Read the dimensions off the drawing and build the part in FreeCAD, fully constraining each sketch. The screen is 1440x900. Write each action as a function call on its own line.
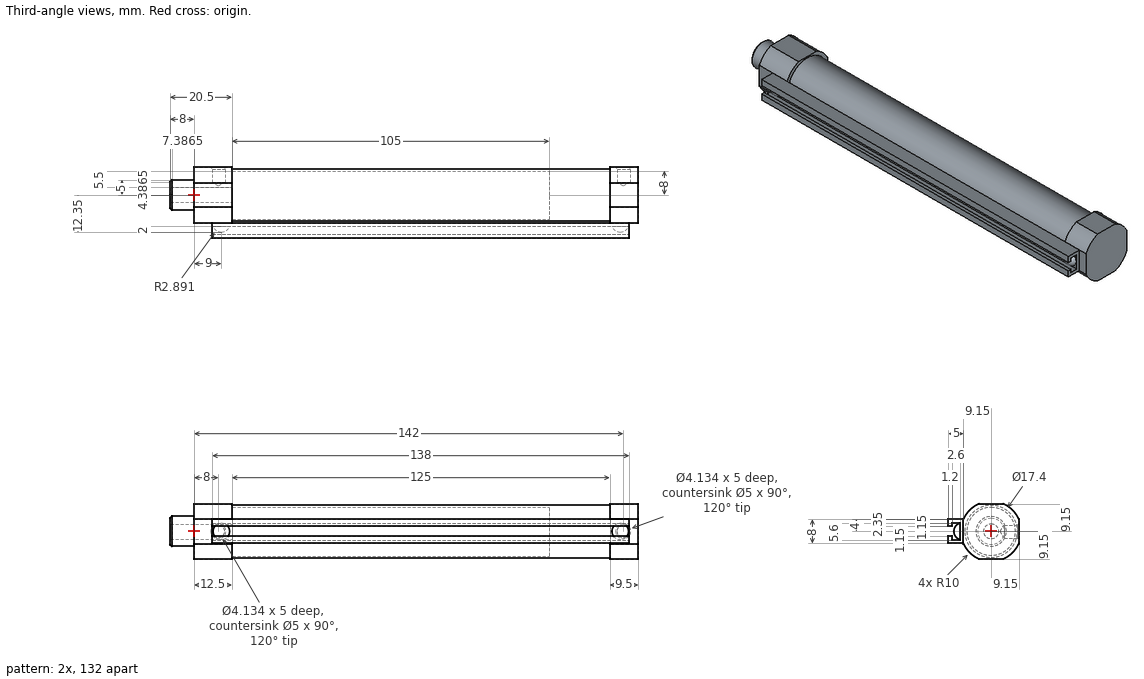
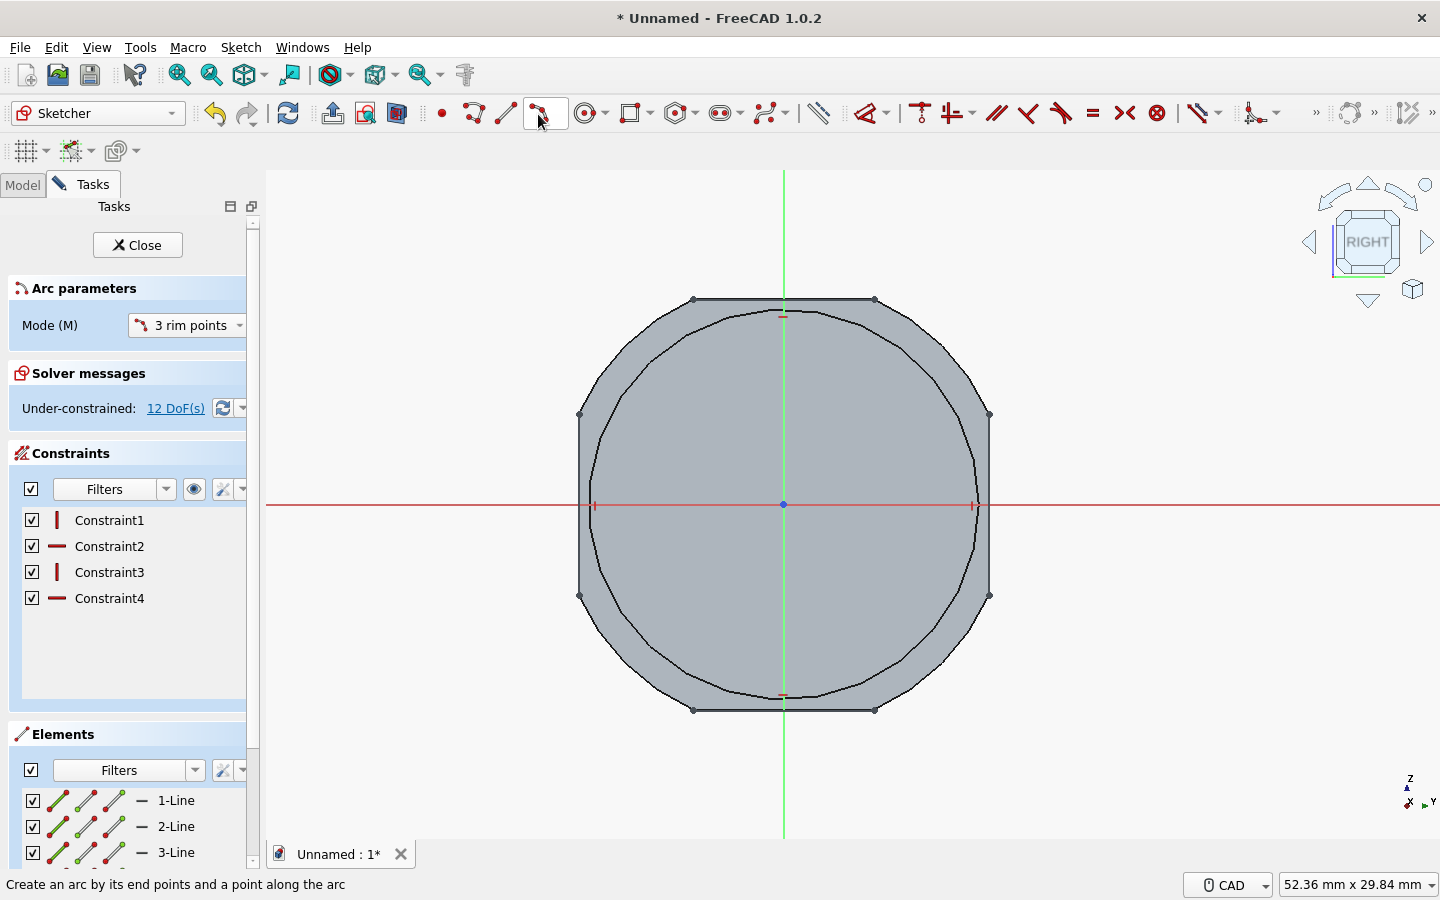
click(579, 596)
click(693, 711)
click(625, 663)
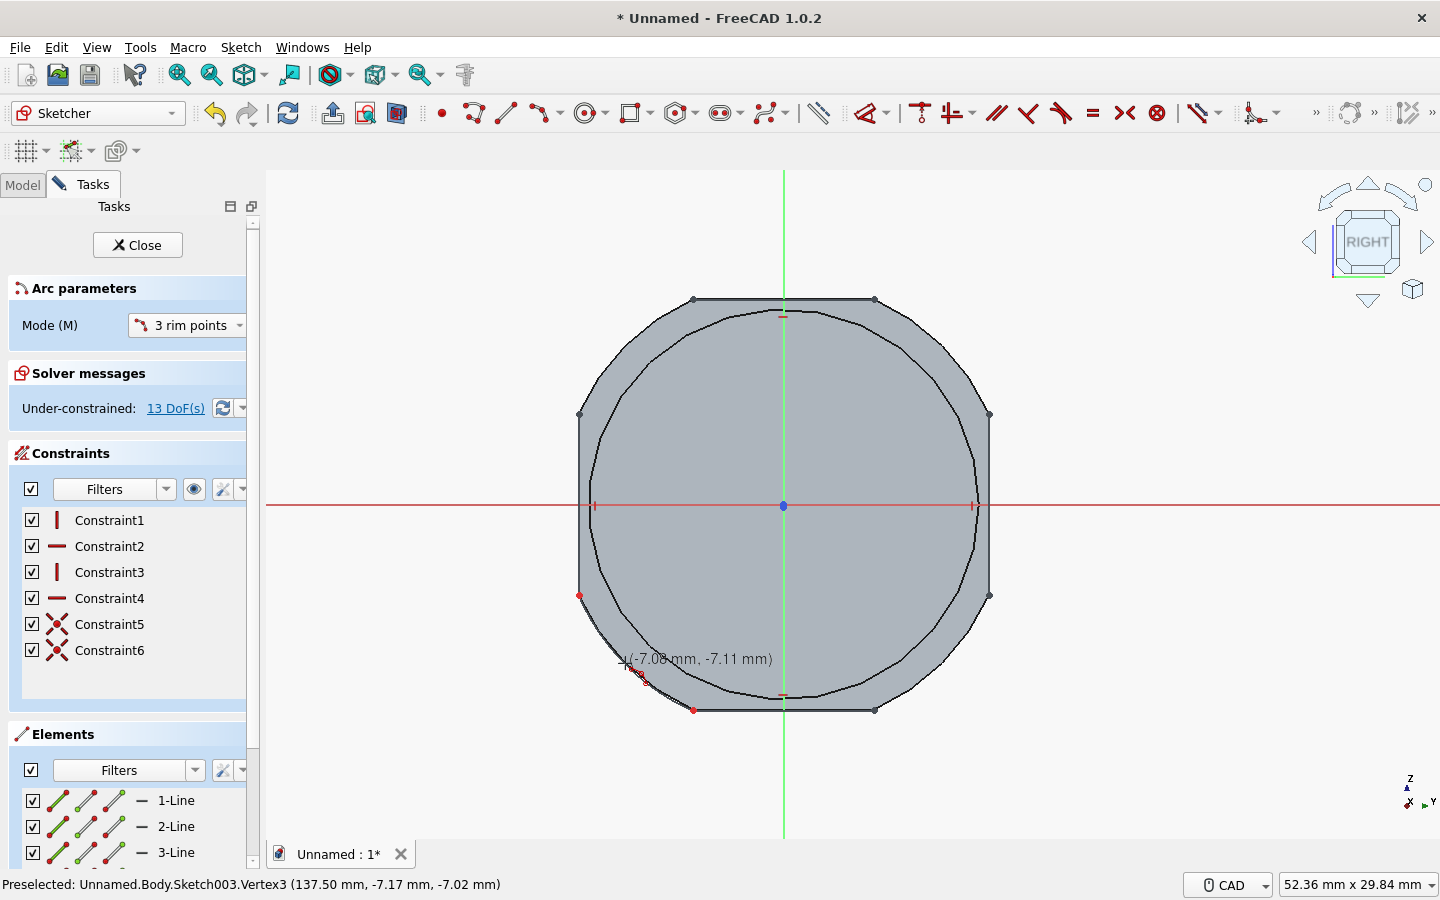
click(874, 711)
click(989, 596)
click(942, 663)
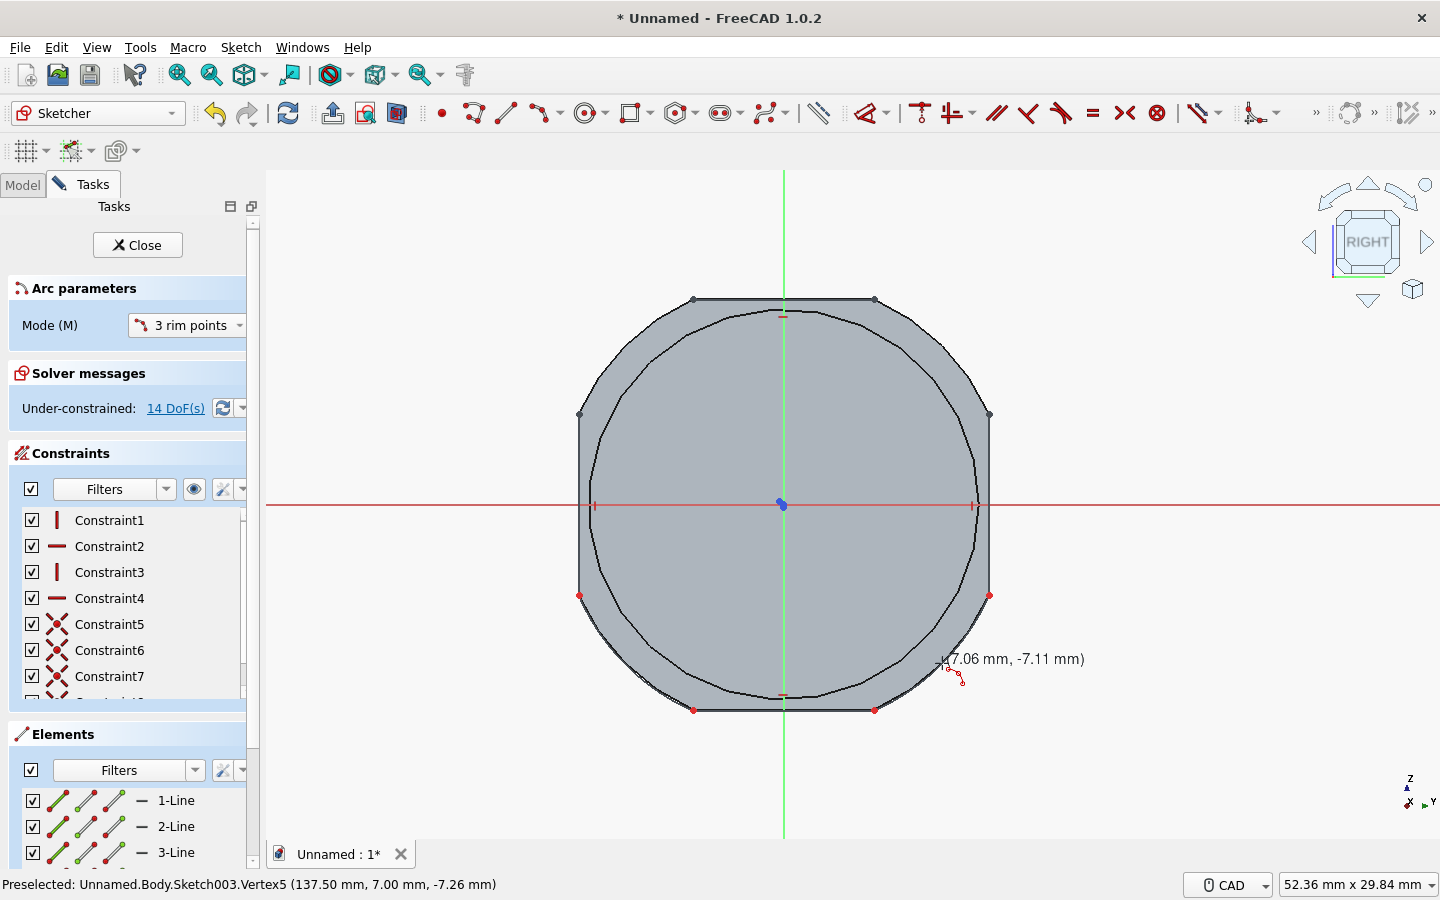
click(989, 415)
click(874, 300)
click(942, 346)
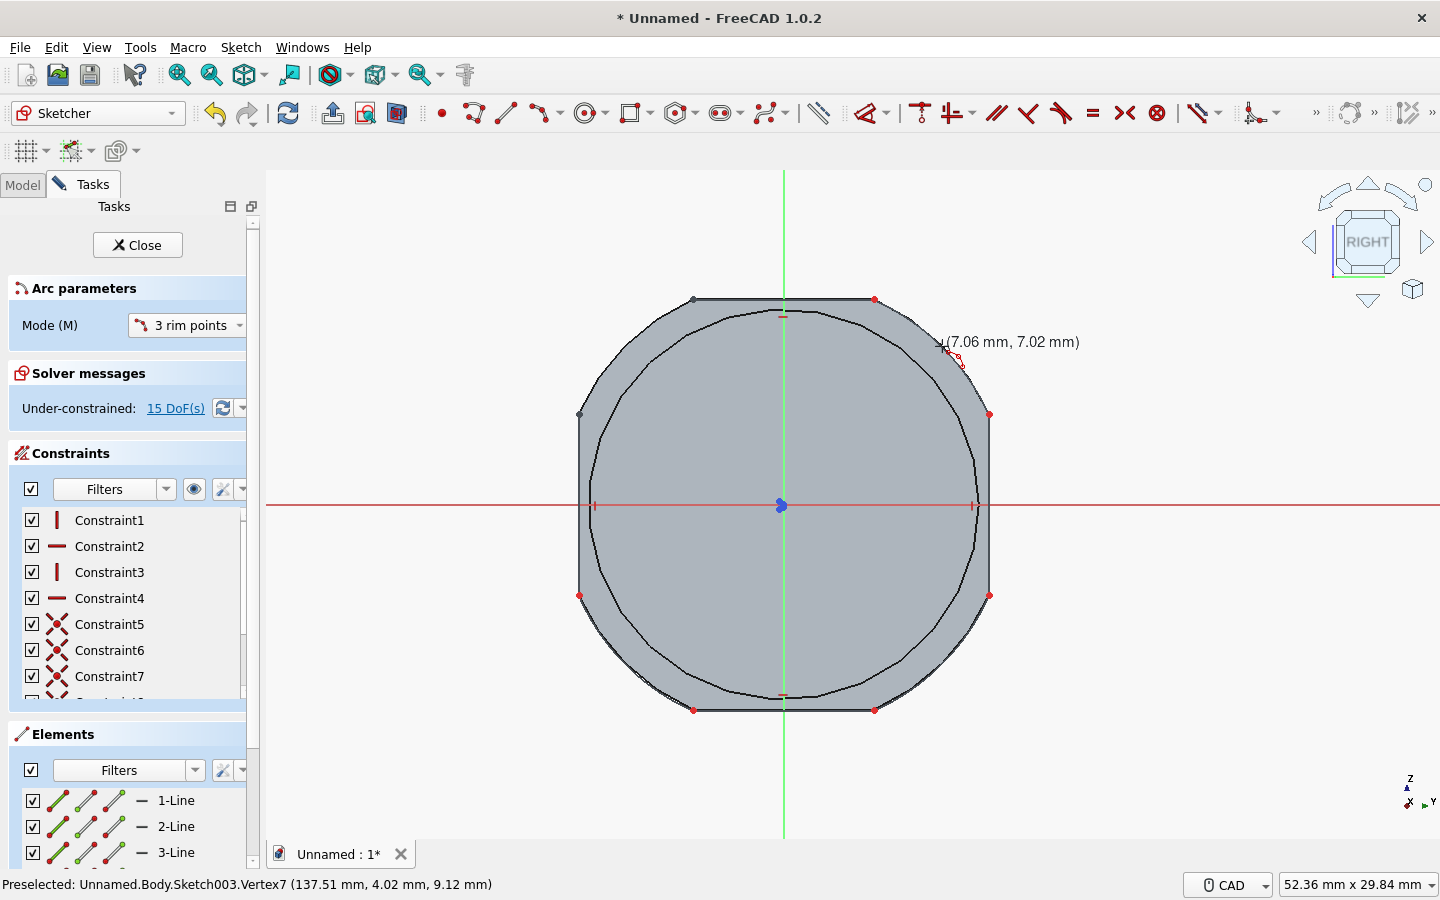
click(693, 300)
click(579, 415)
click(625, 346)
key(Escape)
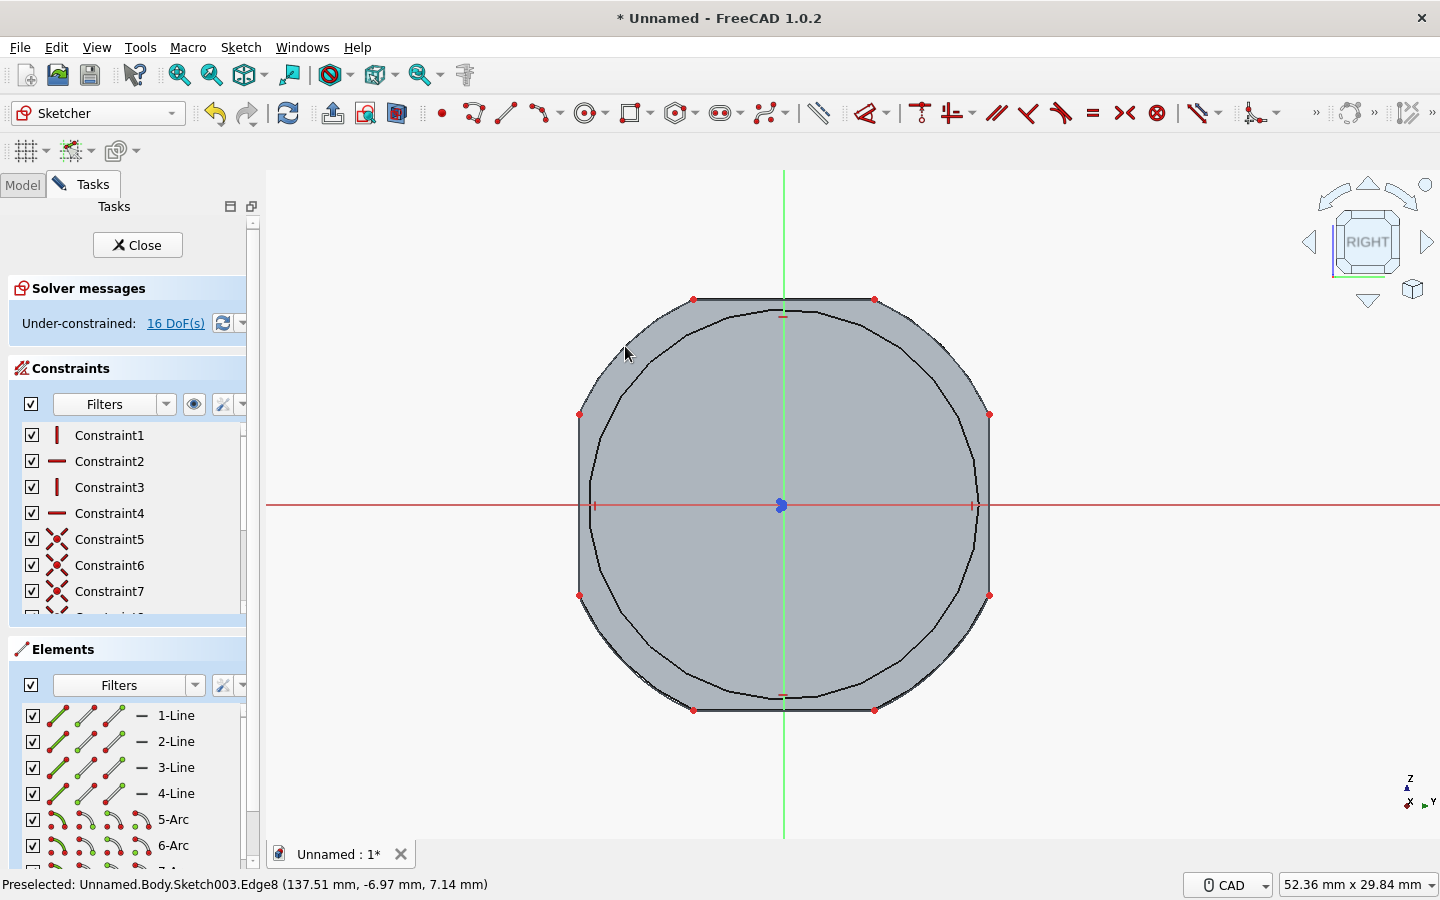
click(604, 639)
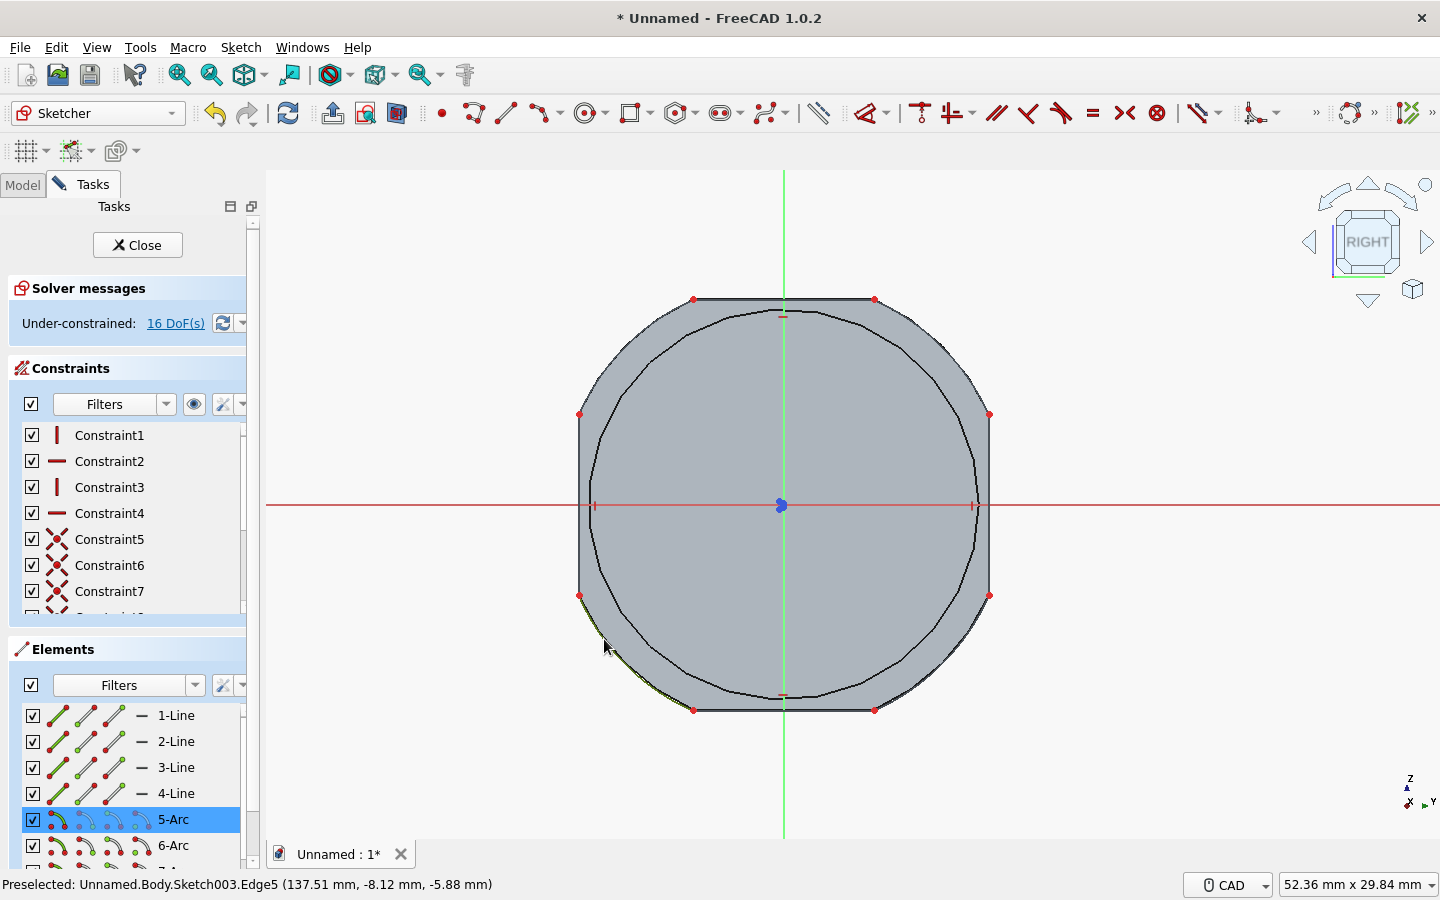
click(917, 686)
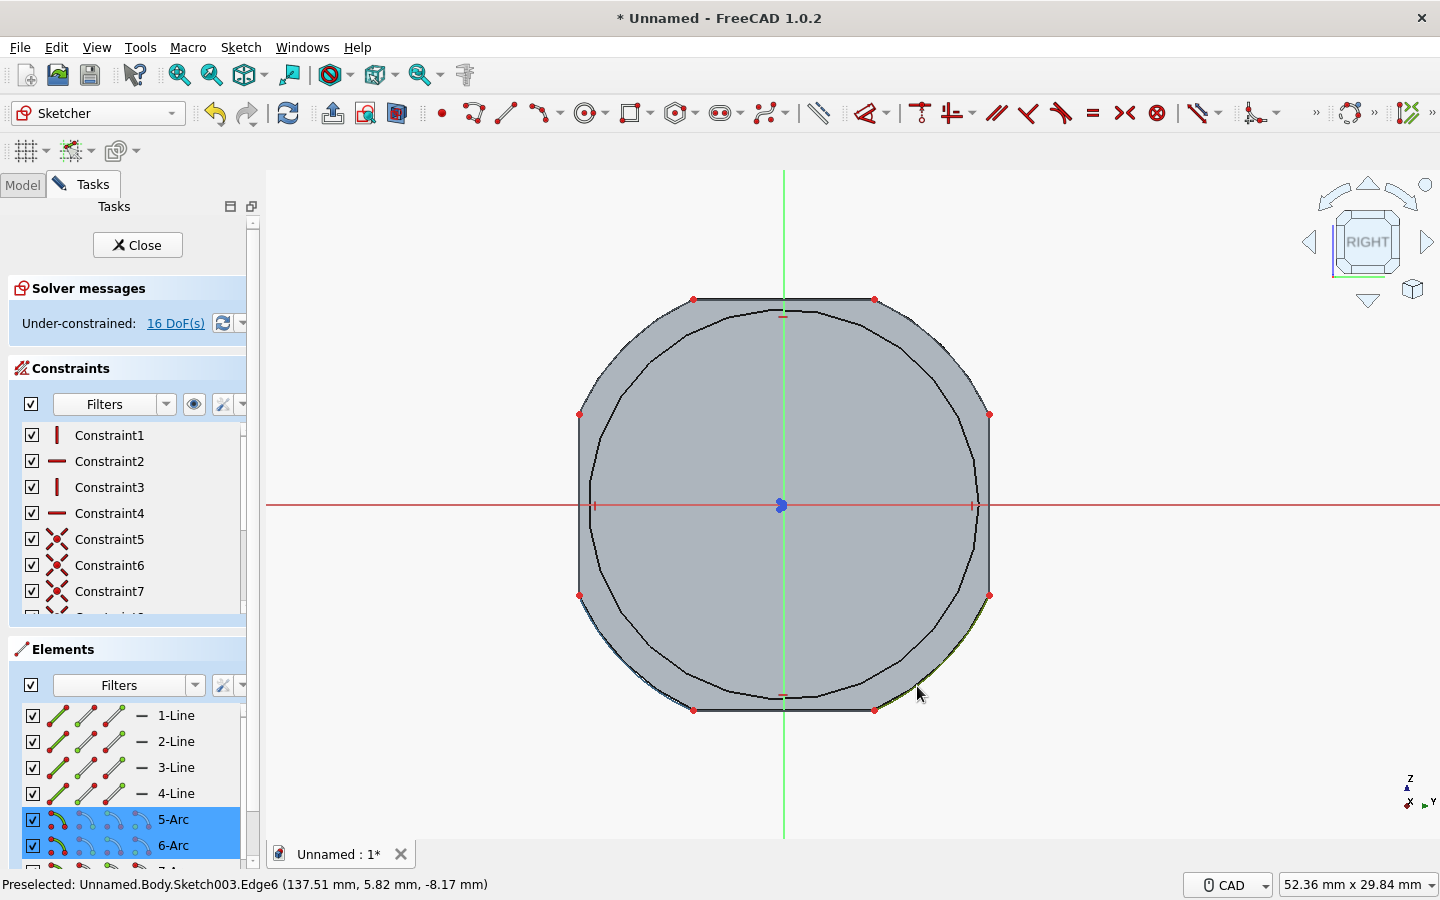
click(920, 114)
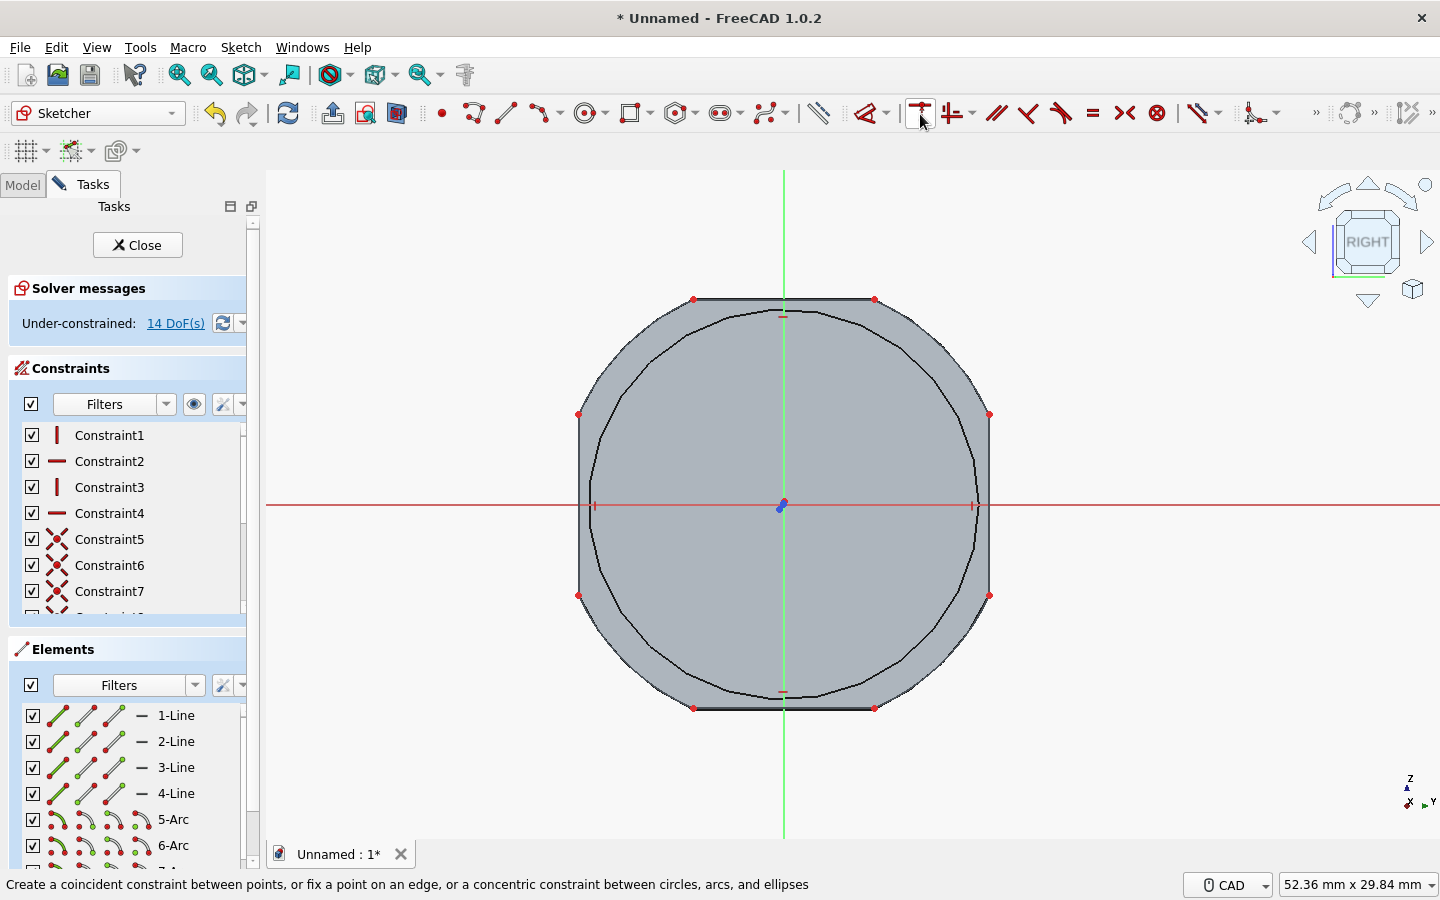
click(604, 638)